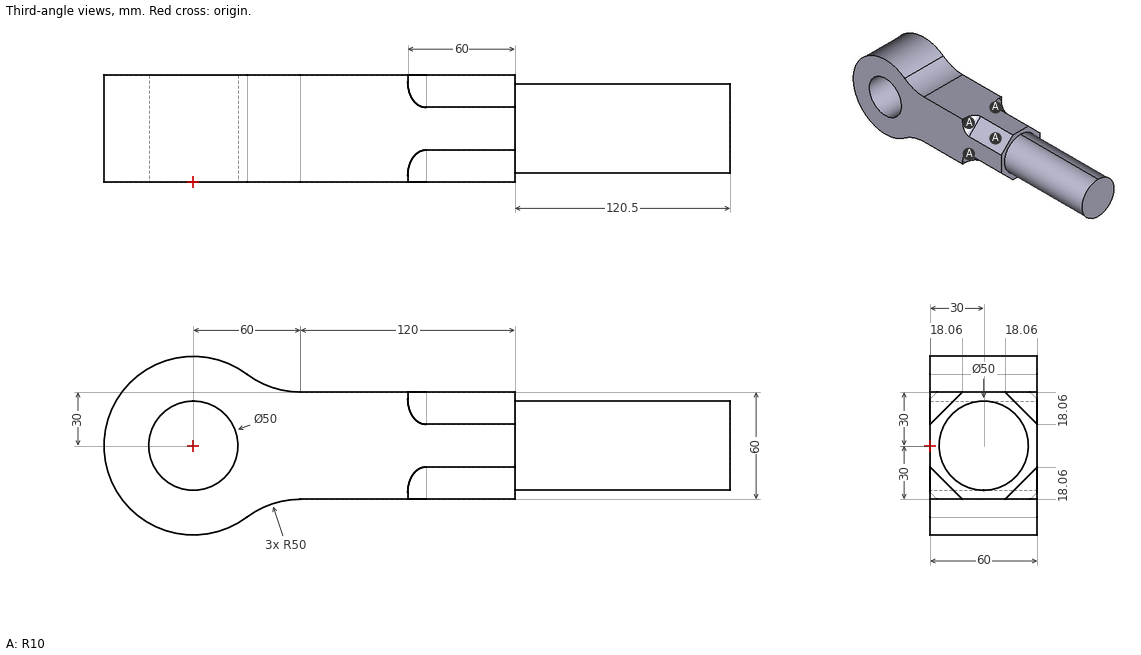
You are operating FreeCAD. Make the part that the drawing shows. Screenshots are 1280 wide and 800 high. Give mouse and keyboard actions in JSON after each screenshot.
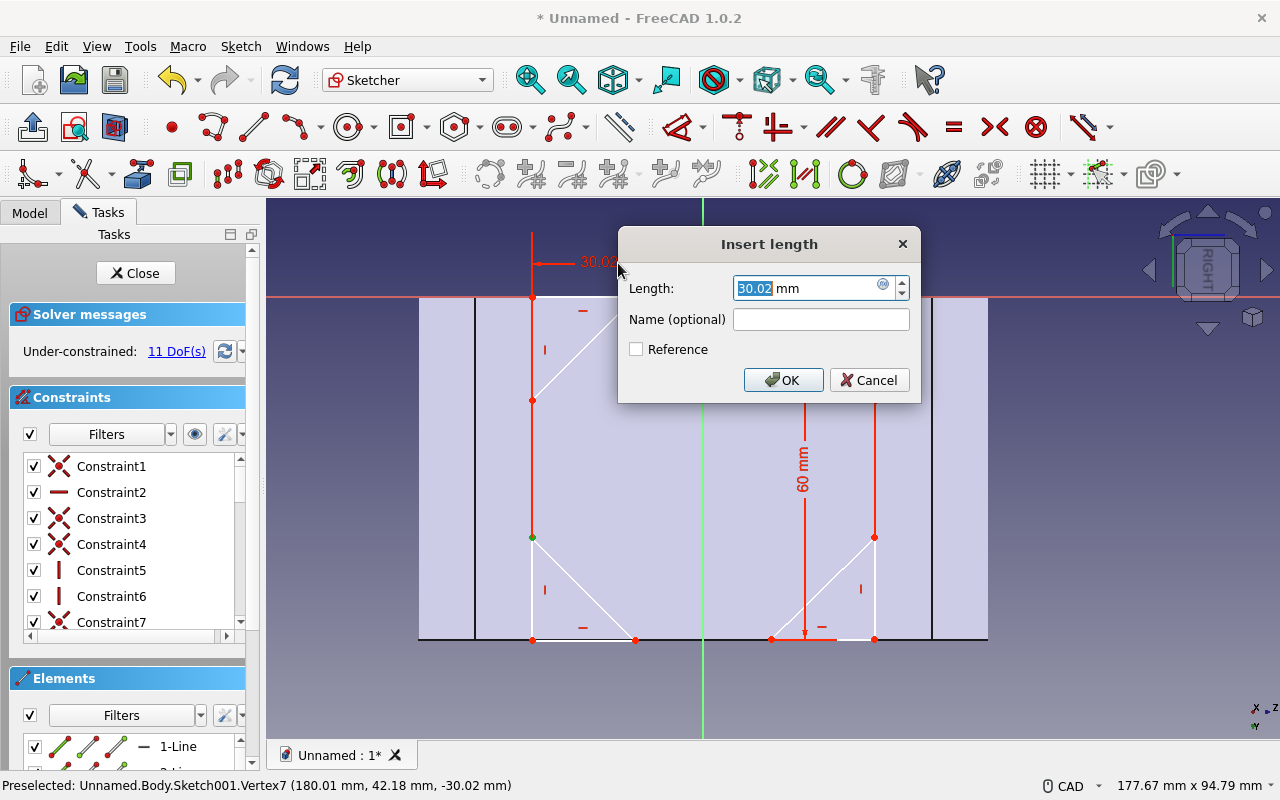
{"action": "type", "text": "30"}
{"action": "key", "text": "Return"}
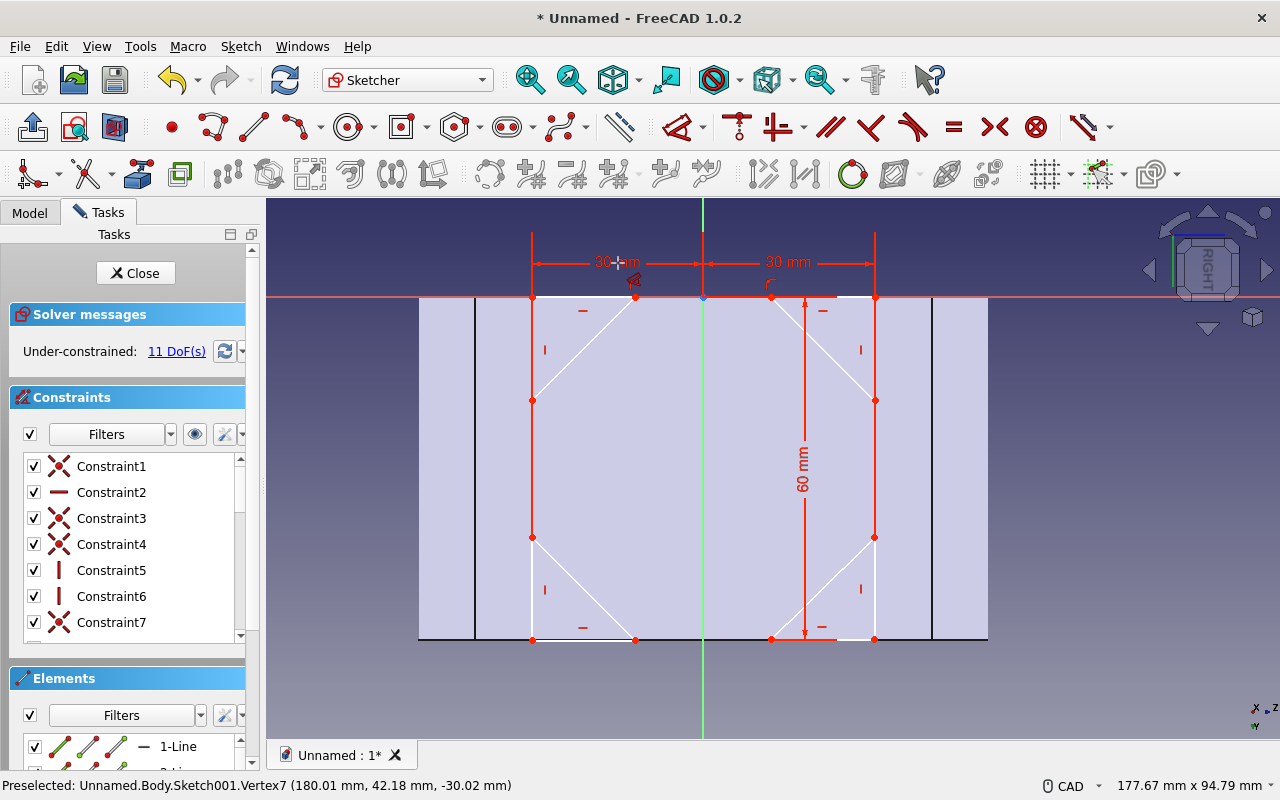
{"action": "left_click", "coordinate": [532, 641]}
{"action": "left_click", "coordinate": [498, 469]}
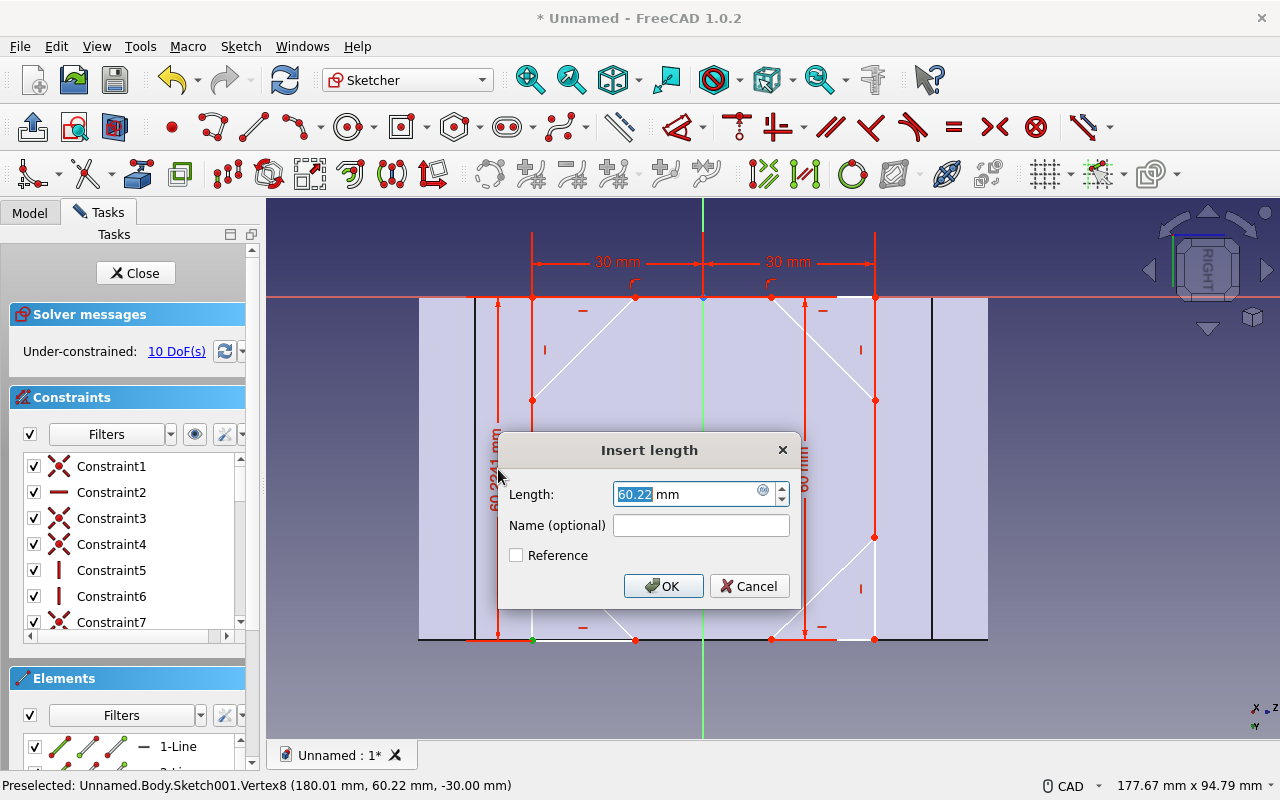
{"action": "type", "text": "60"}
{"action": "key", "text": "Return"}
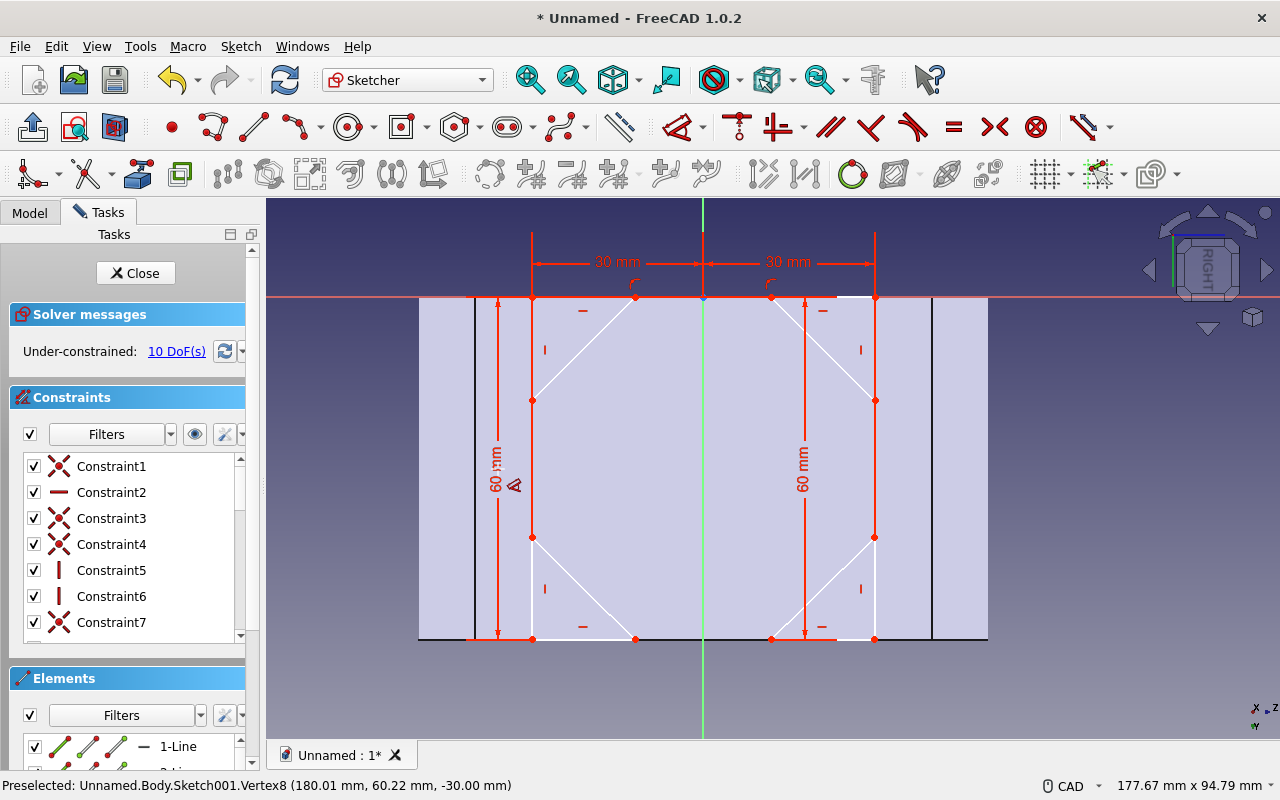
{"action": "left_click", "coordinate": [875, 401]}
{"action": "left_click", "coordinate": [789, 435]}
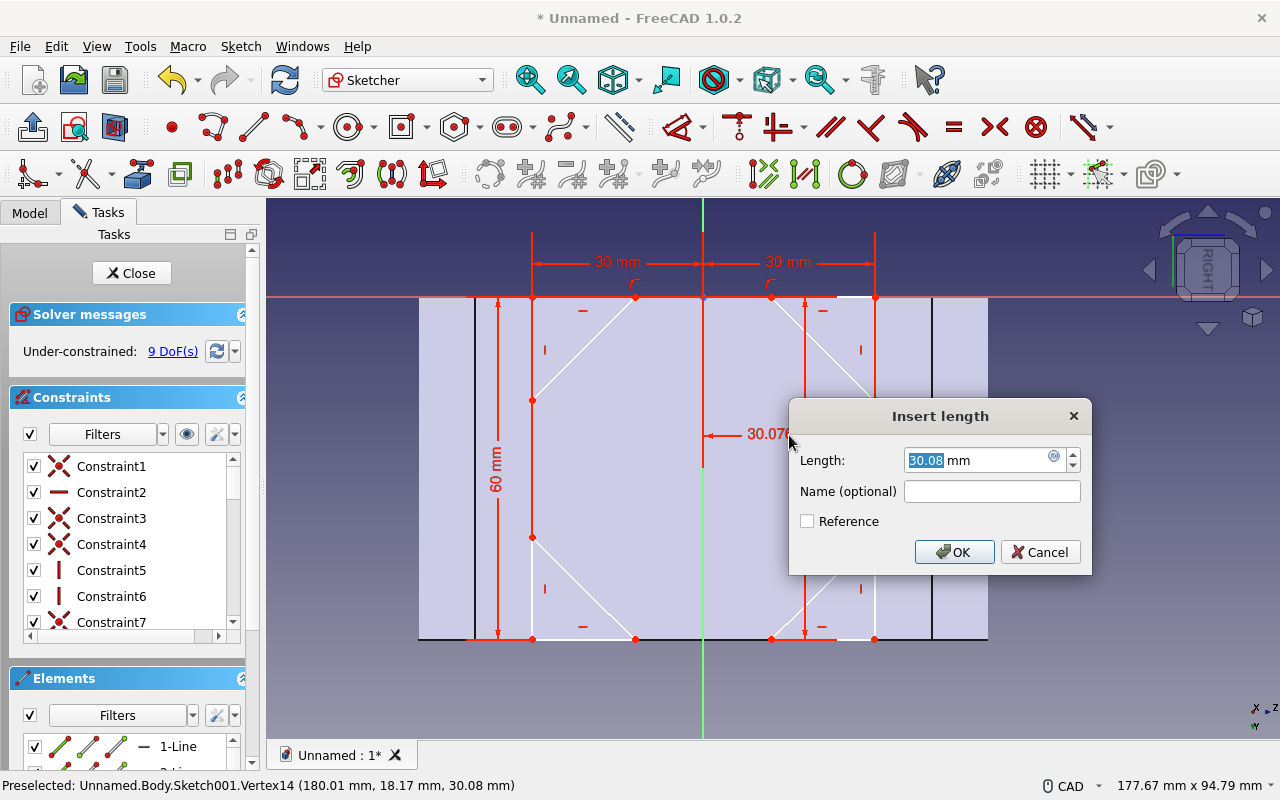
{"action": "type", "text": "30"}
{"action": "key", "text": "Return"}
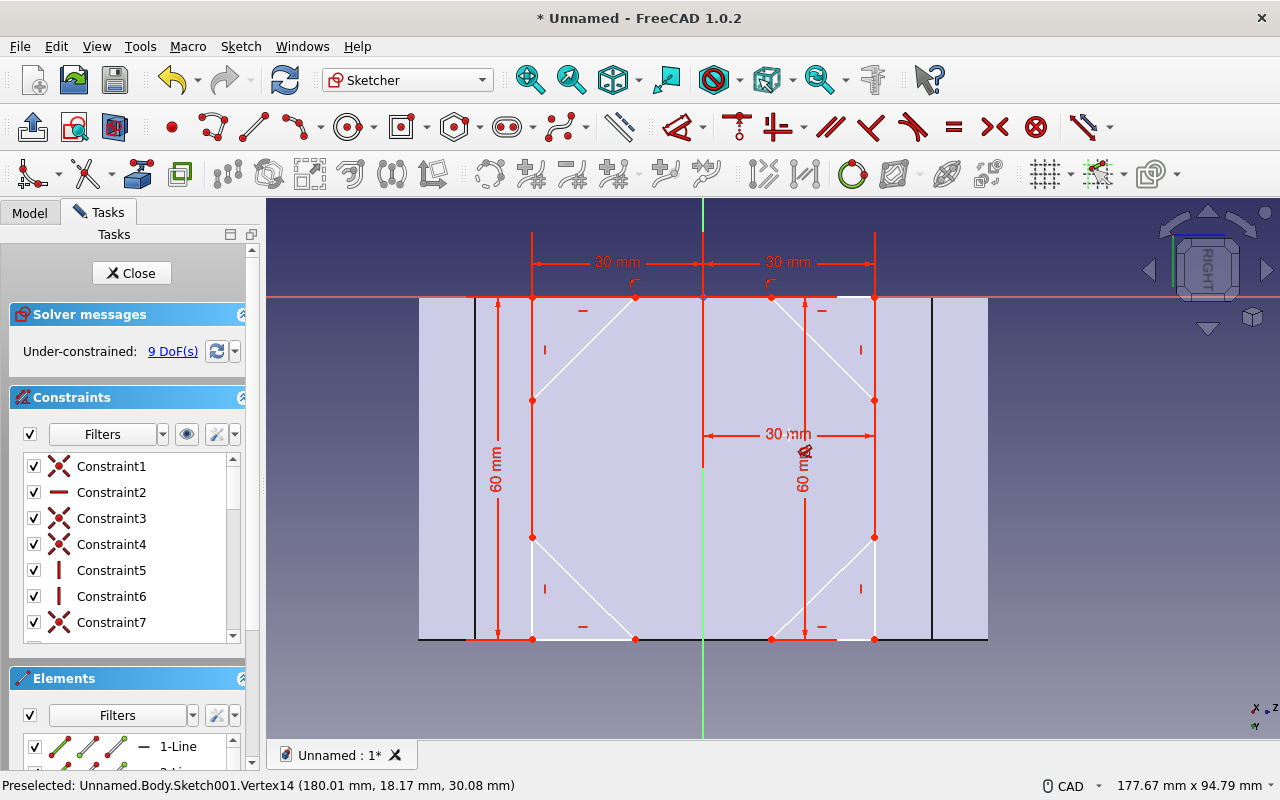
{"action": "left_click", "coordinate": [532, 297]}
{"action": "left_click", "coordinate": [578, 331]}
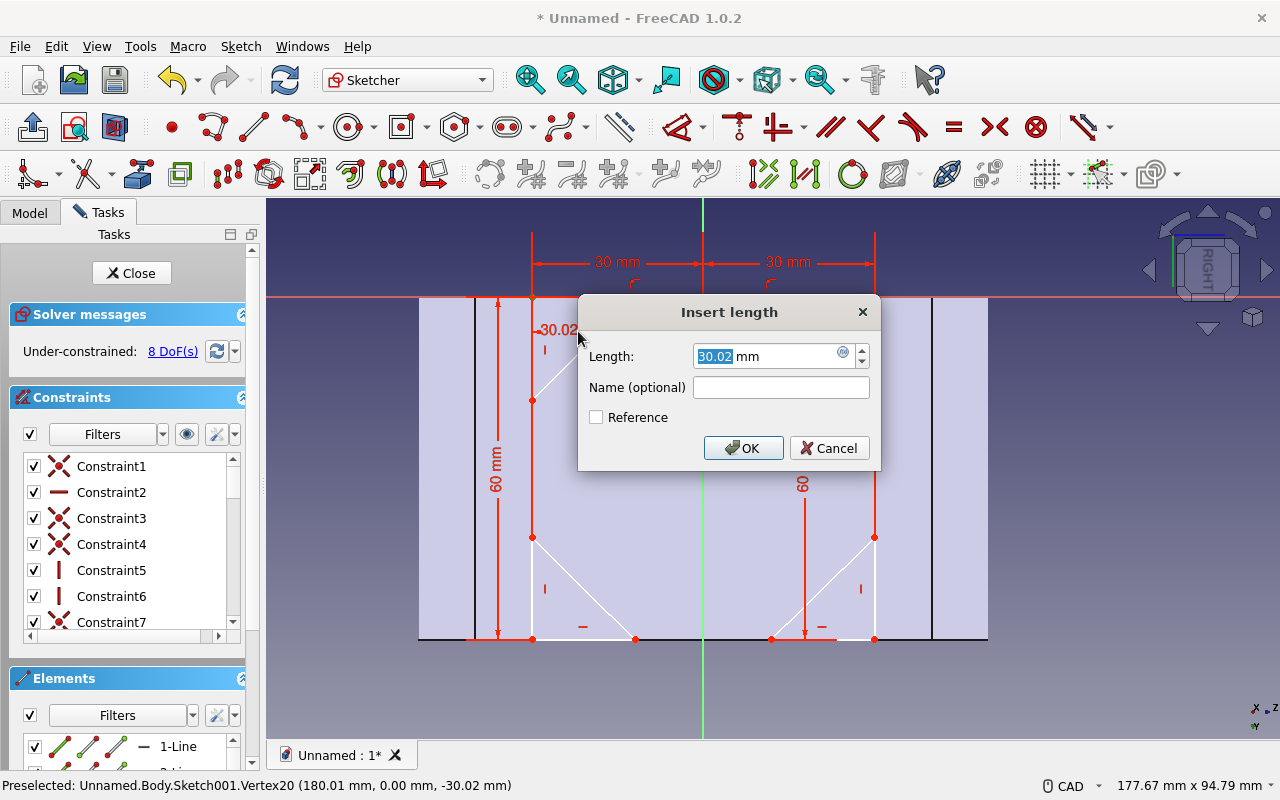
{"action": "type", "text": "30"}
{"action": "key", "text": "Return"}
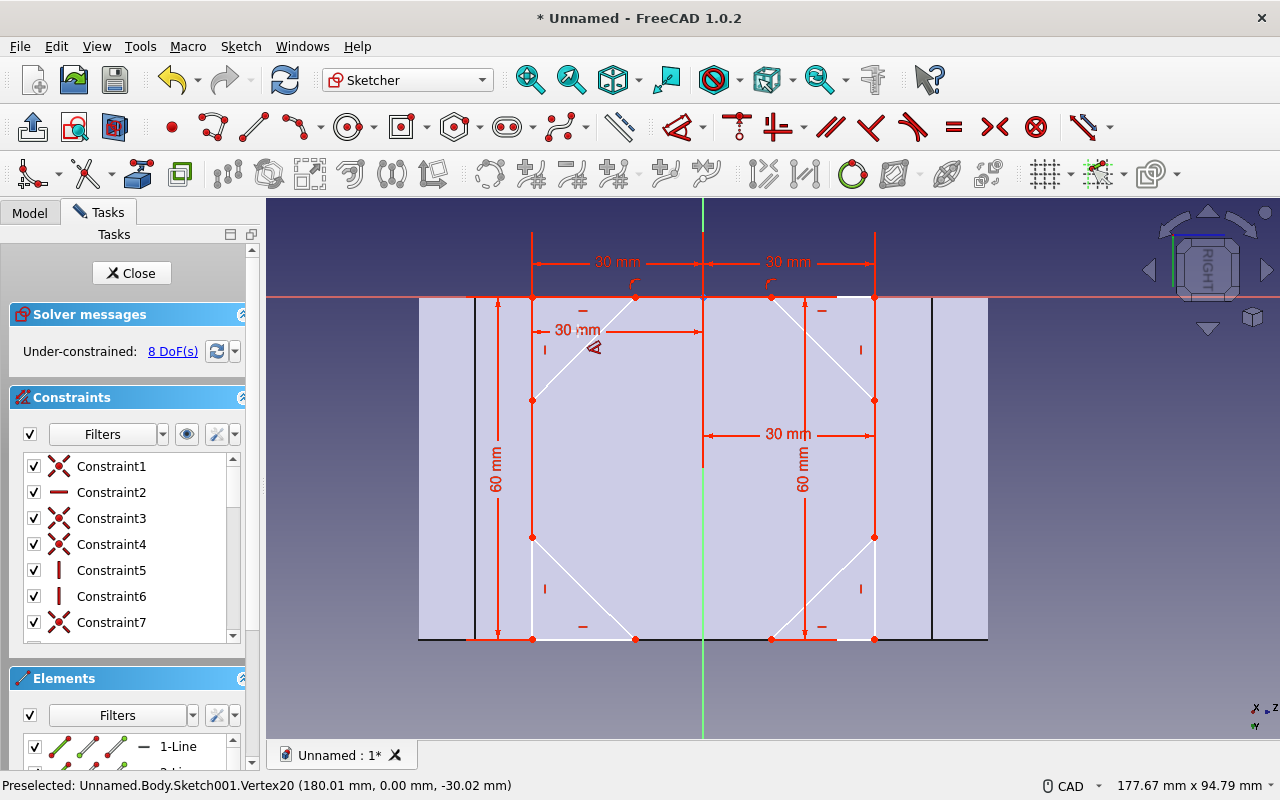
{"action": "left_click", "coordinate": [802, 640]}
{"action": "left_click", "coordinate": [823, 674]}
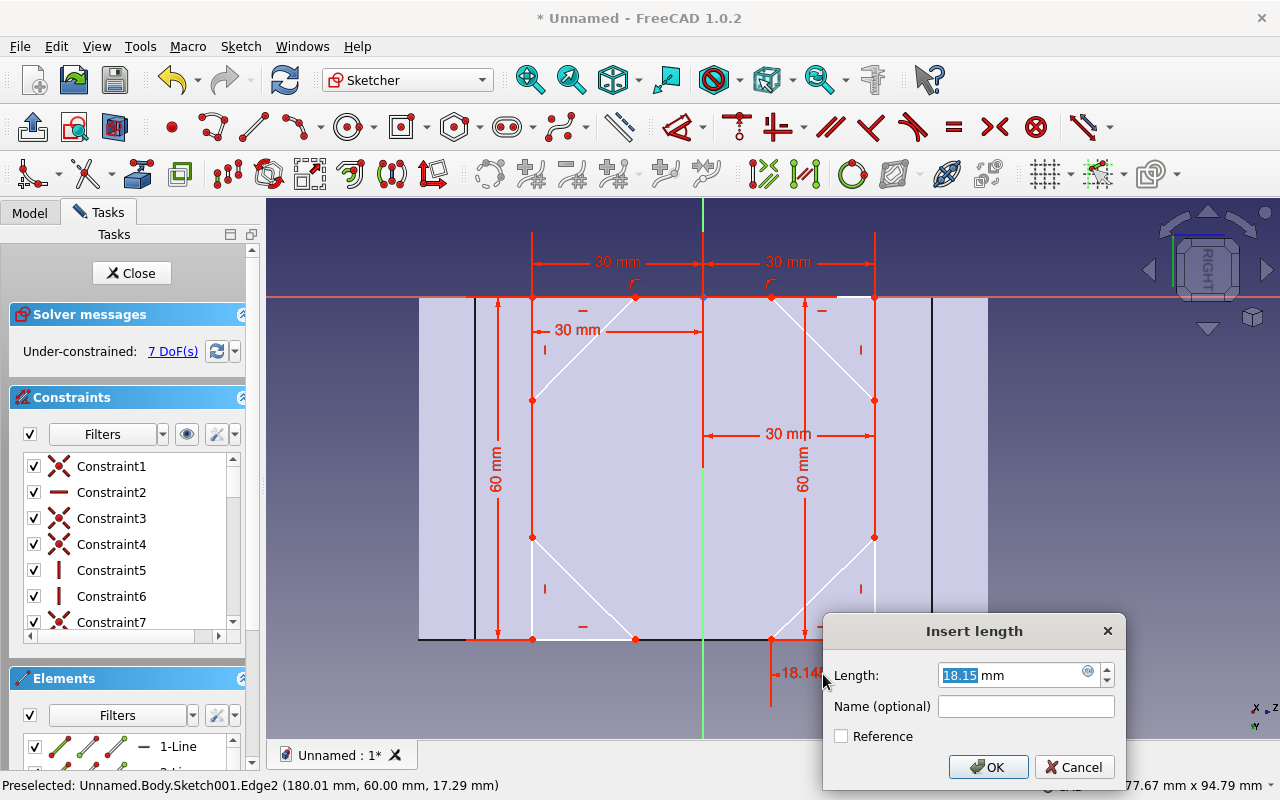
{"action": "type", "text": "18.06"}
{"action": "key", "text": "Return"}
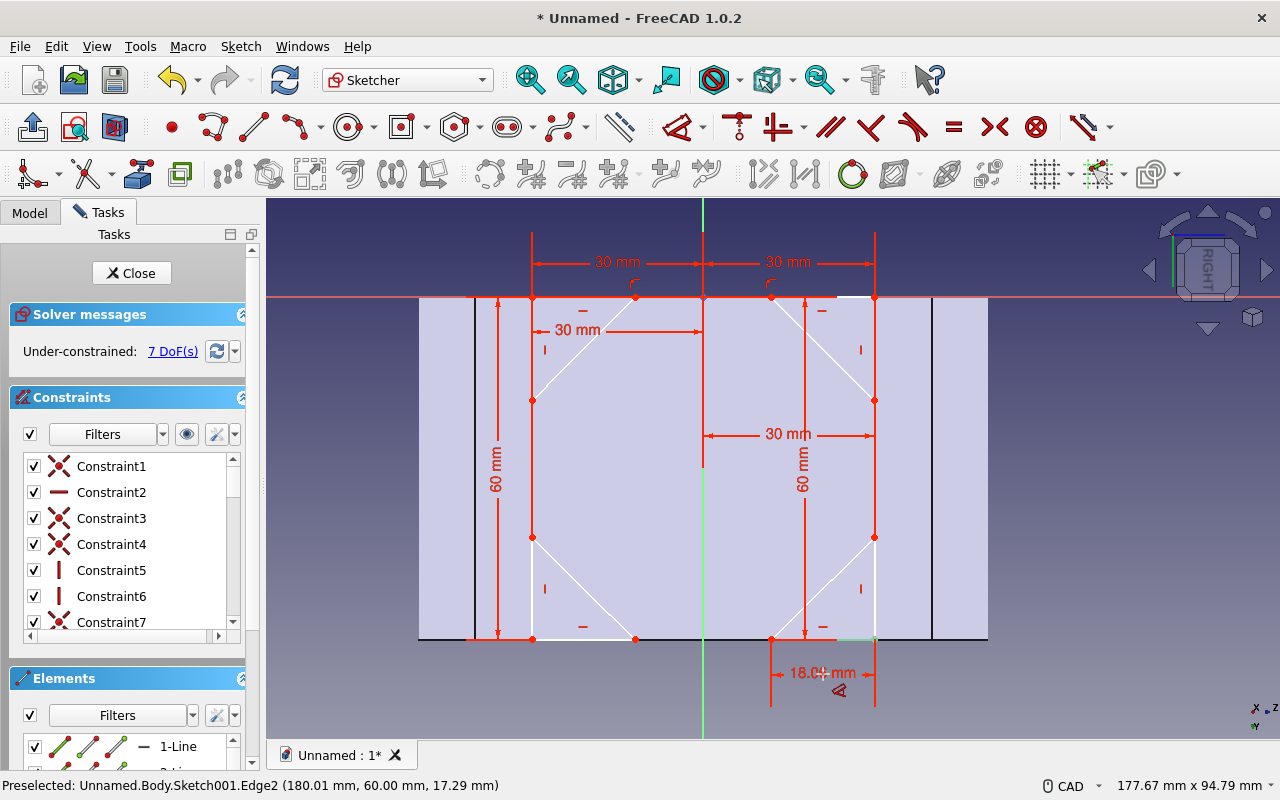
{"action": "left_click", "coordinate": [875, 609]}
{"action": "left_click", "coordinate": [909, 589]}